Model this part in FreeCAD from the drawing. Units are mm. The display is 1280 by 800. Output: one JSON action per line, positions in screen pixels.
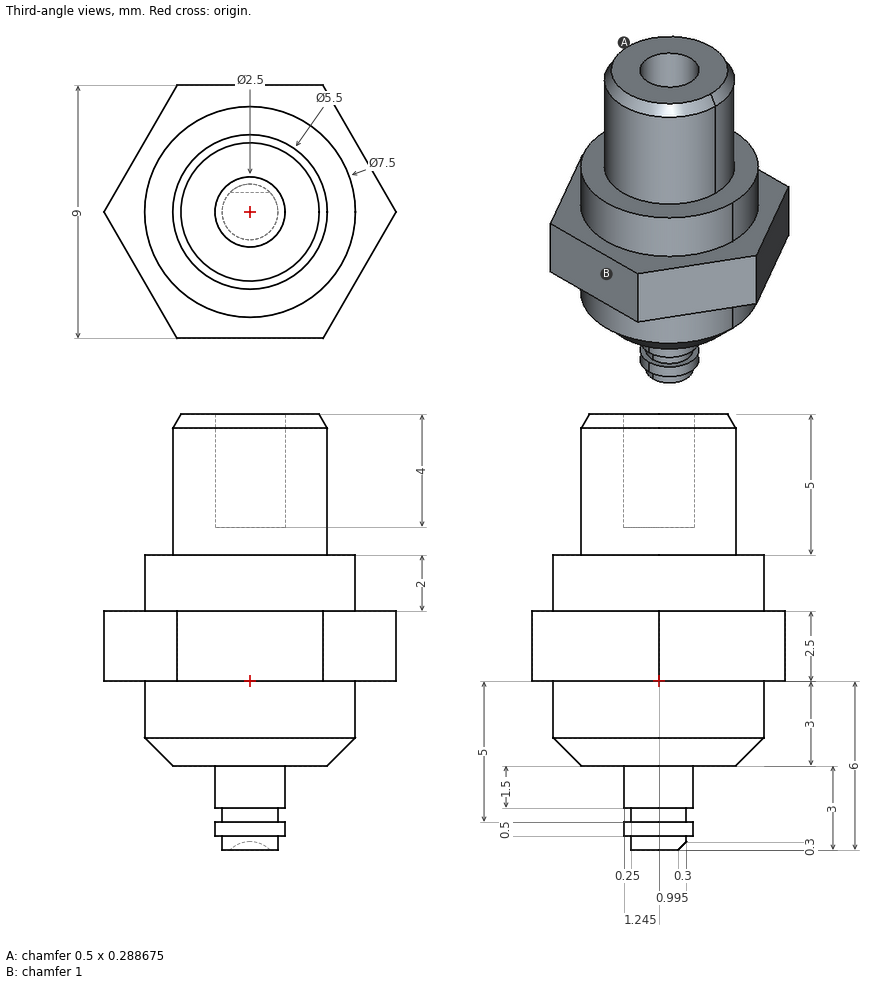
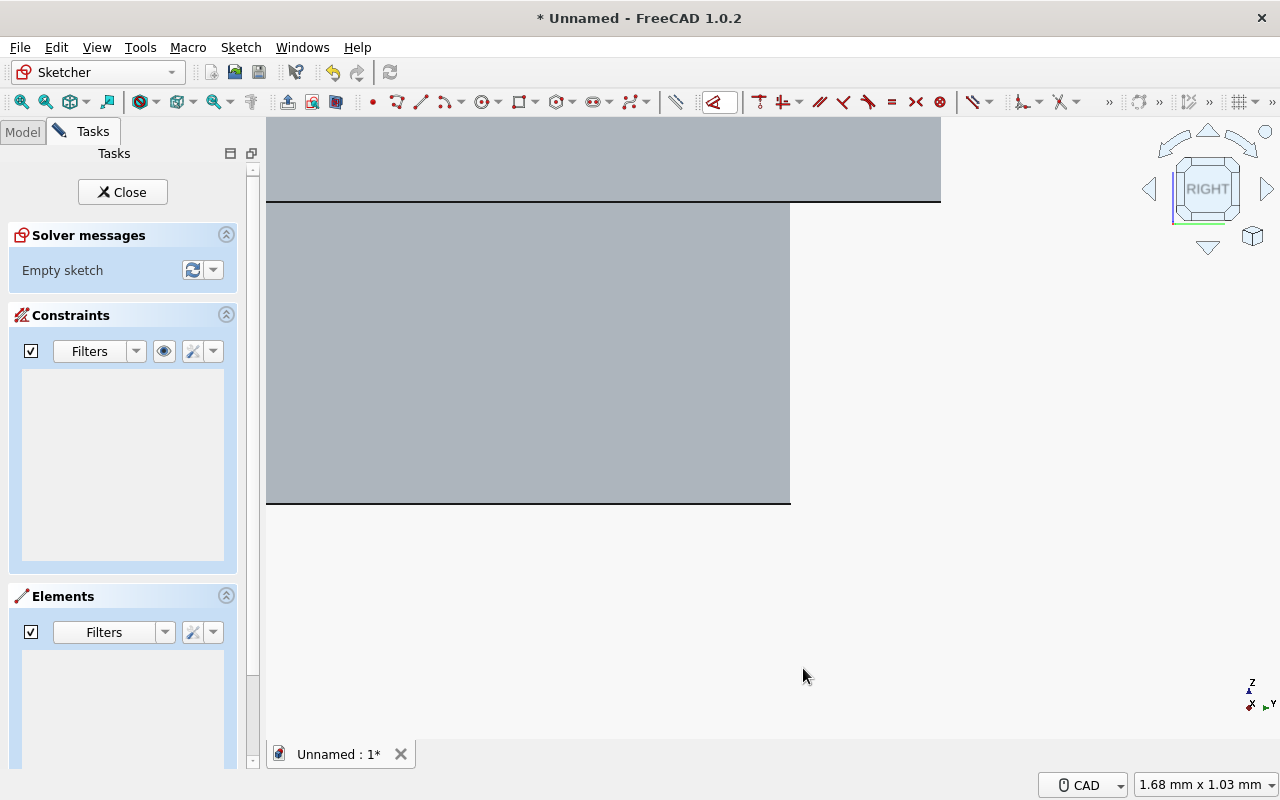
{"action": "scroll", "coordinate": [696, 401], "scroll_direction": "up", "scroll_amount": 4}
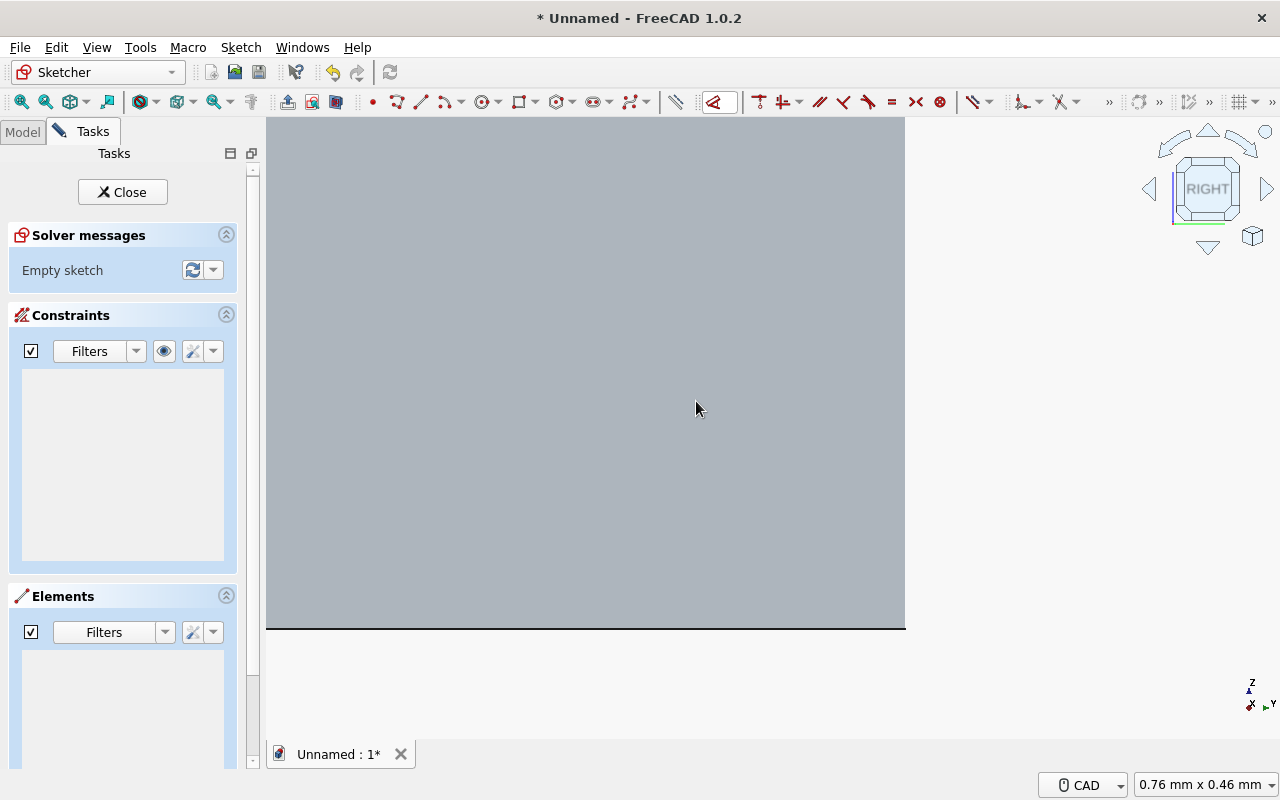
{"action": "key", "text": "g m"}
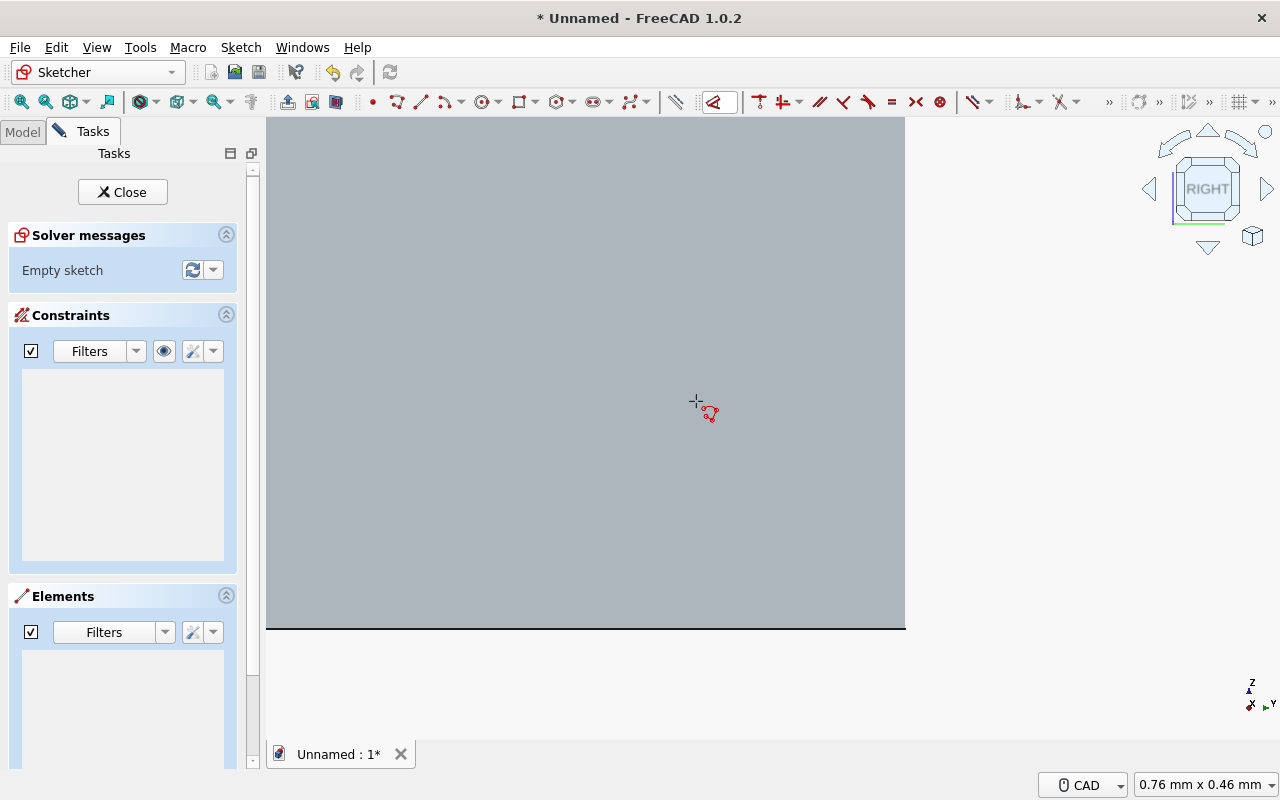
{"action": "left_click", "coordinate": [905, 227]}
{"action": "left_click", "coordinate": [503, 629]}
{"action": "left_click", "coordinate": [905, 629]}
{"action": "left_click", "coordinate": [905, 228]}
{"action": "key", "text": "Escape"}
{"action": "key", "text": "Escape"}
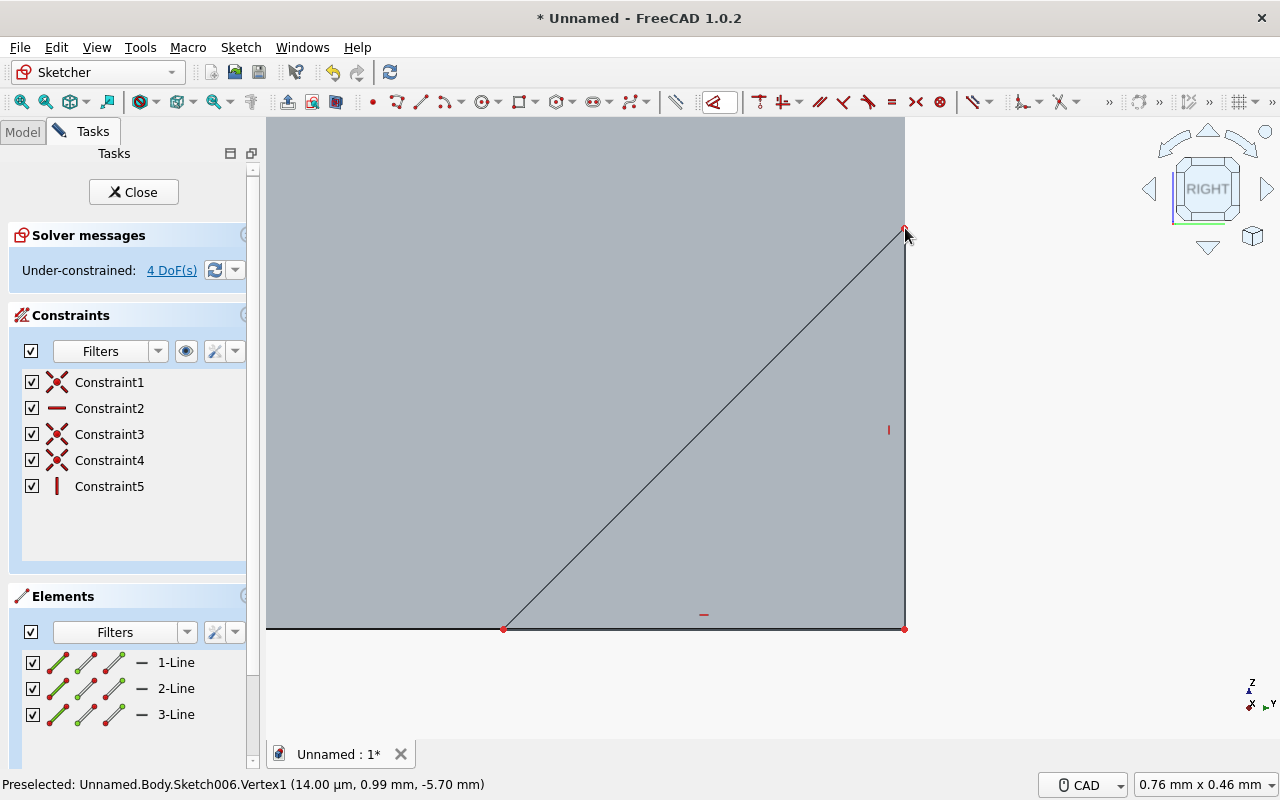
{"action": "left_click", "coordinate": [503, 630]}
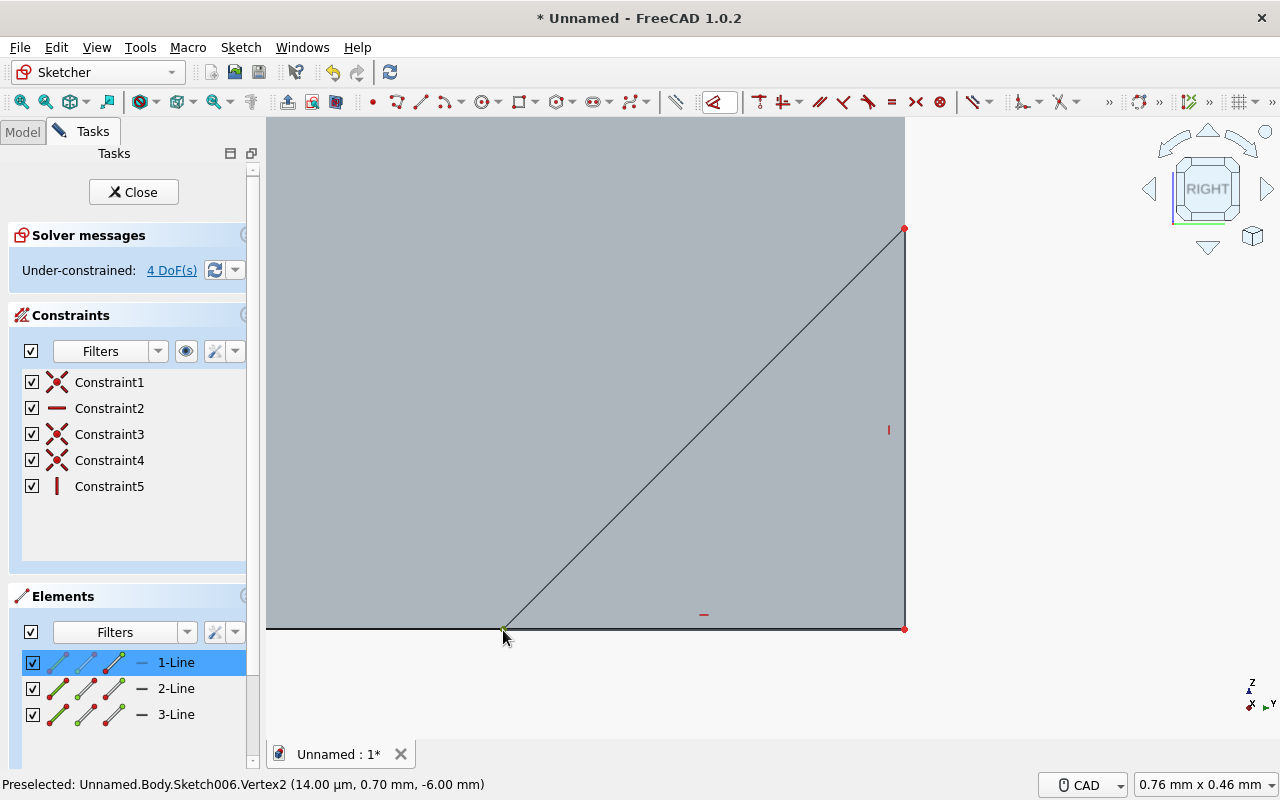
{"action": "key", "text": "i"}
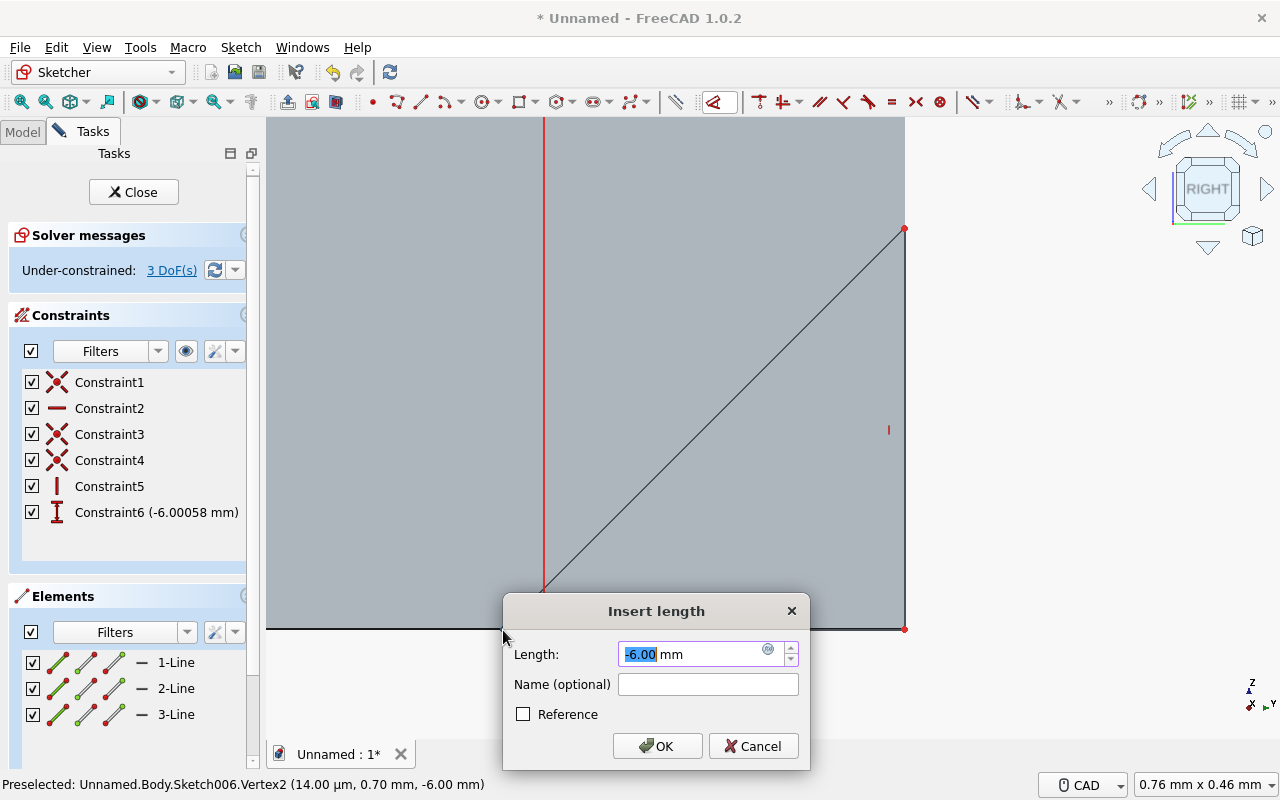
{"action": "type", "text": "-6"}
{"action": "key", "text": "Return"}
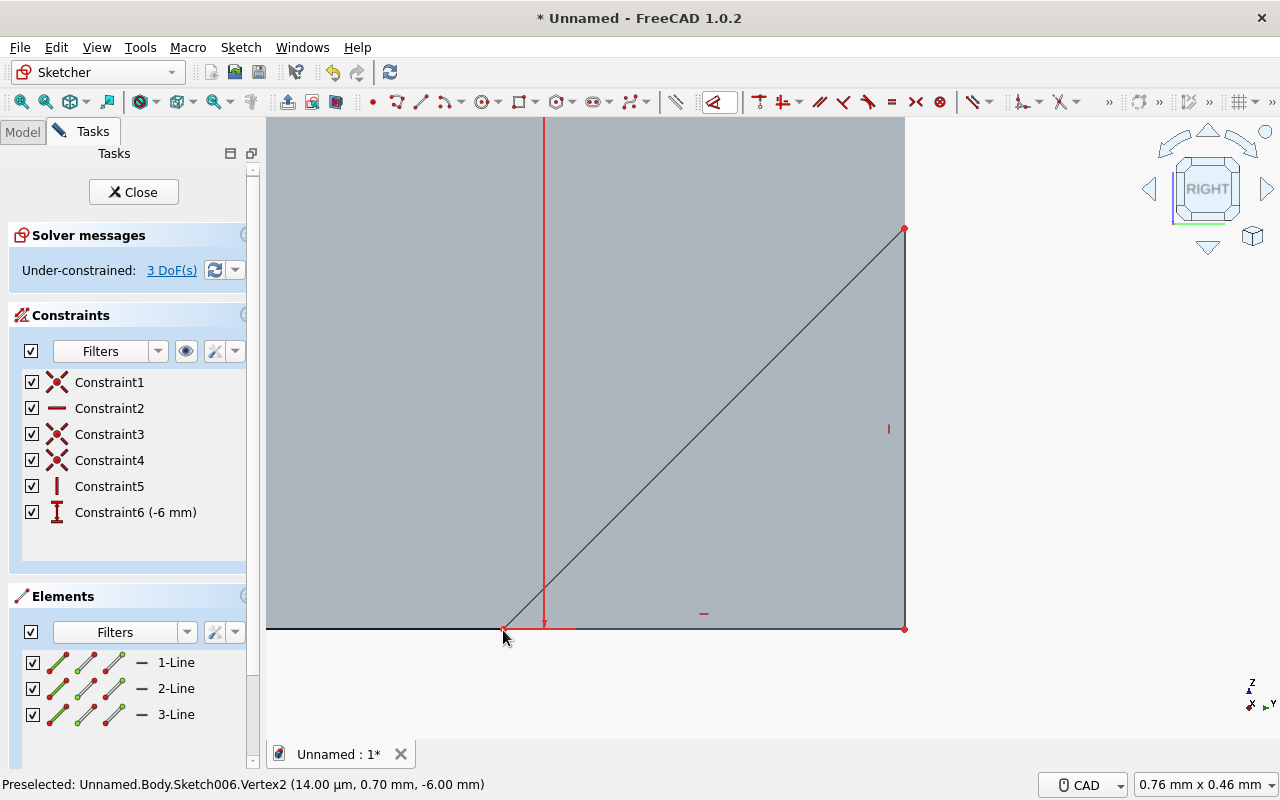
{"action": "left_click", "coordinate": [624, 629]}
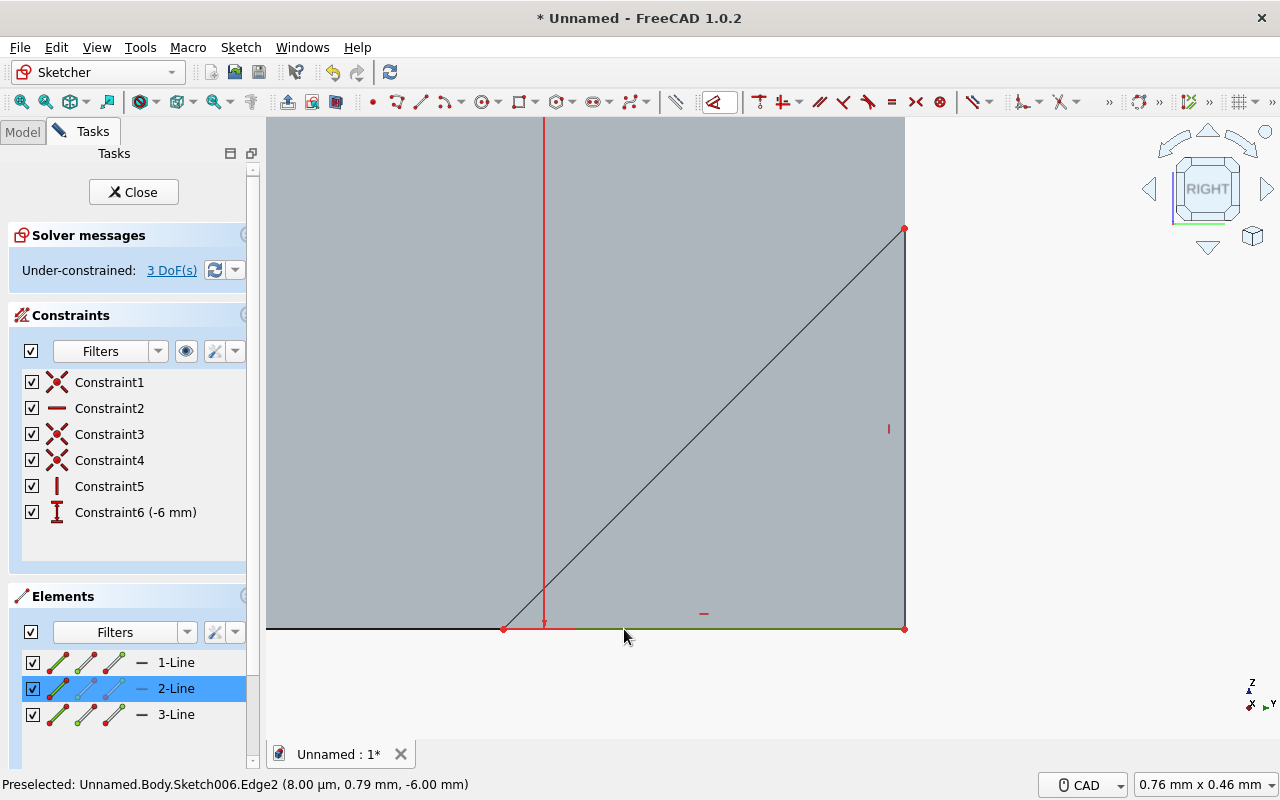
{"action": "key", "text": "l"}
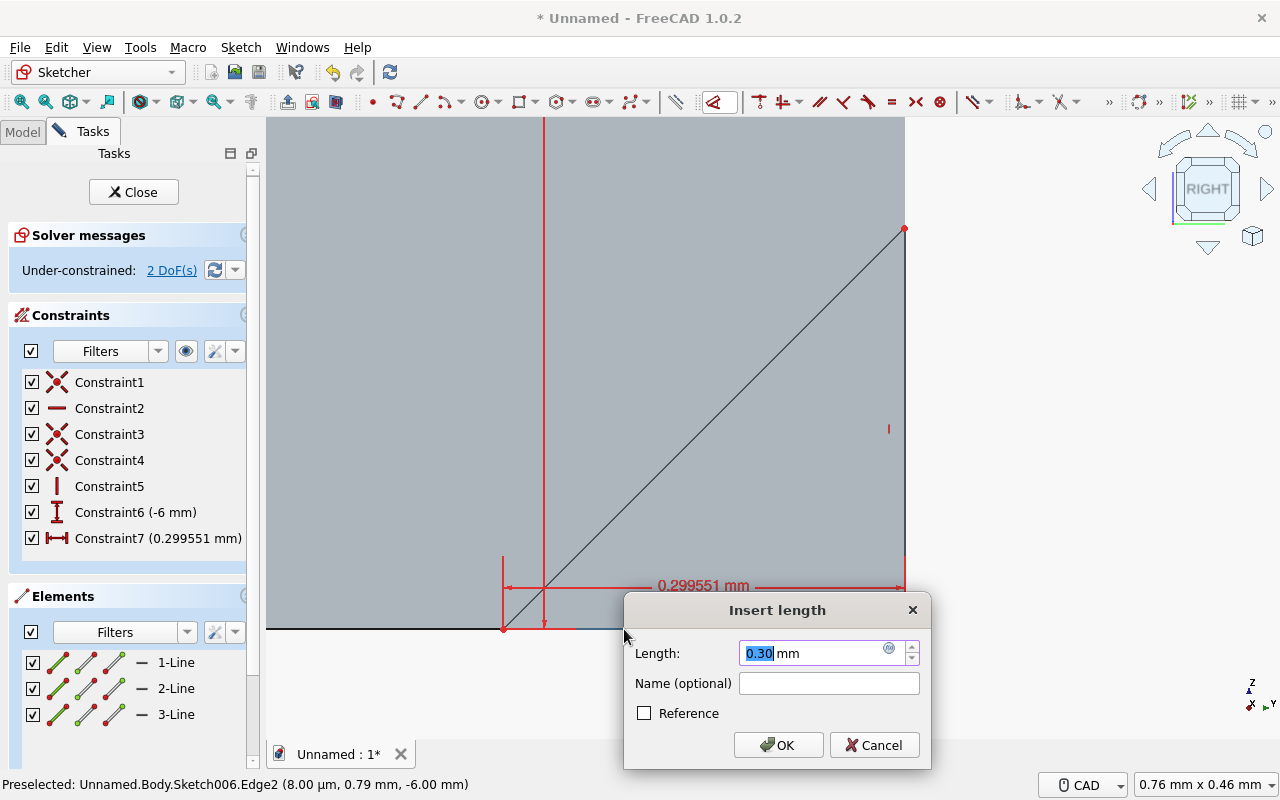
{"action": "type", "text": "0.3"}
{"action": "key", "text": "Return"}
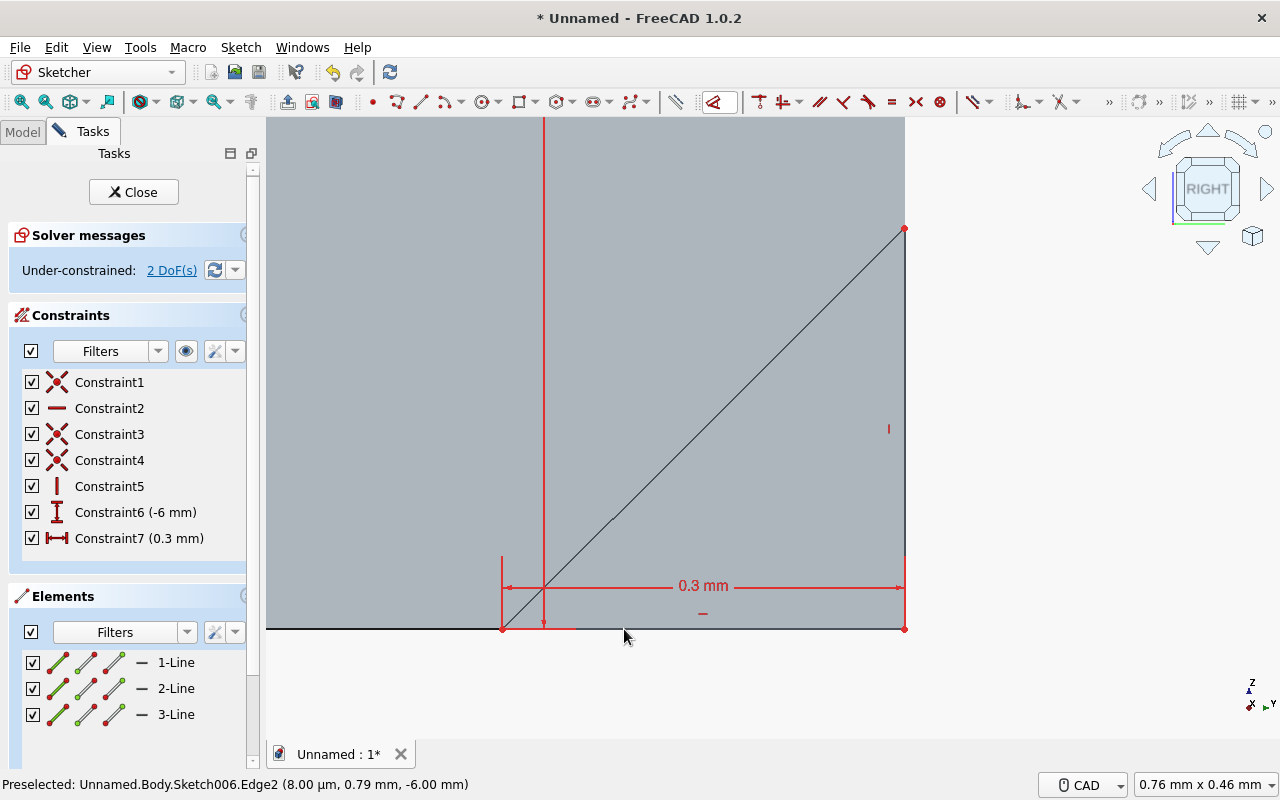
{"action": "left_click", "coordinate": [905, 509]}